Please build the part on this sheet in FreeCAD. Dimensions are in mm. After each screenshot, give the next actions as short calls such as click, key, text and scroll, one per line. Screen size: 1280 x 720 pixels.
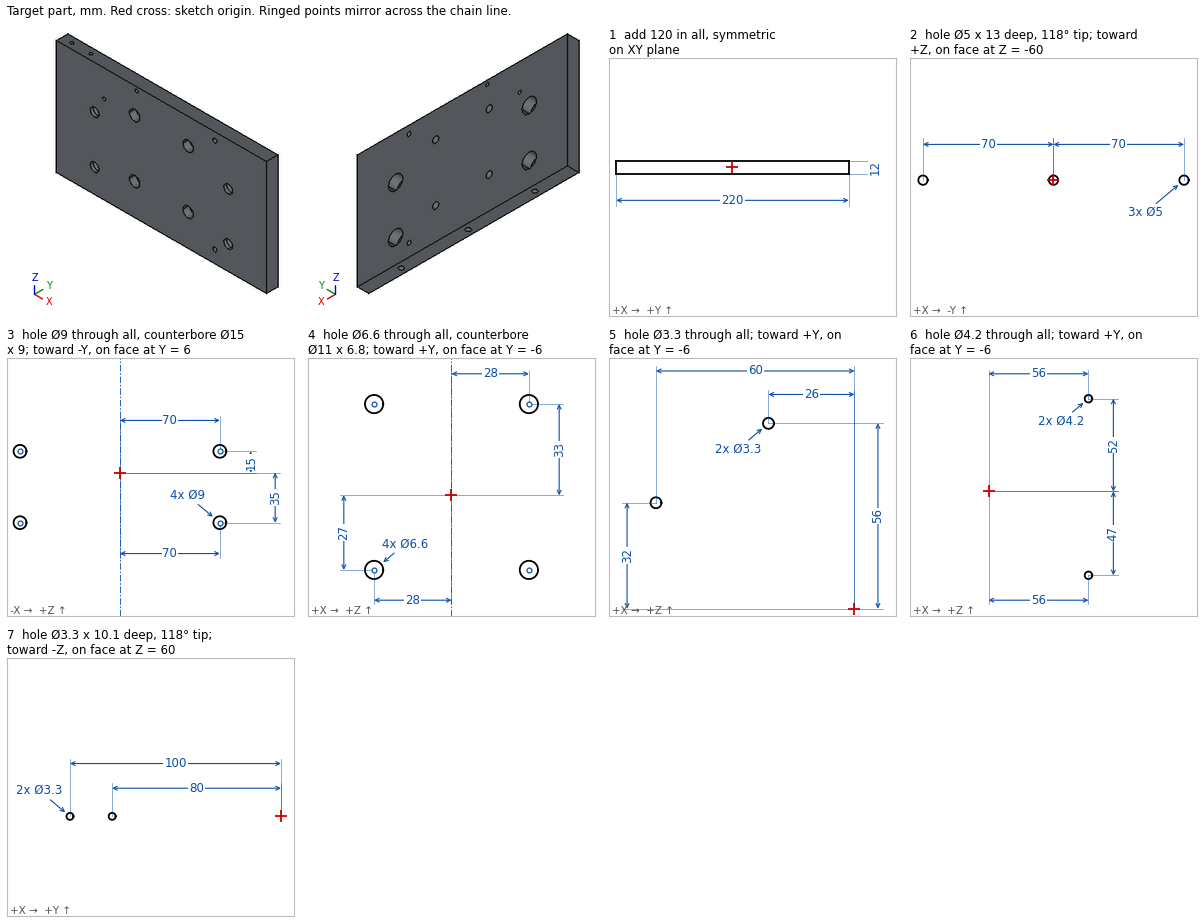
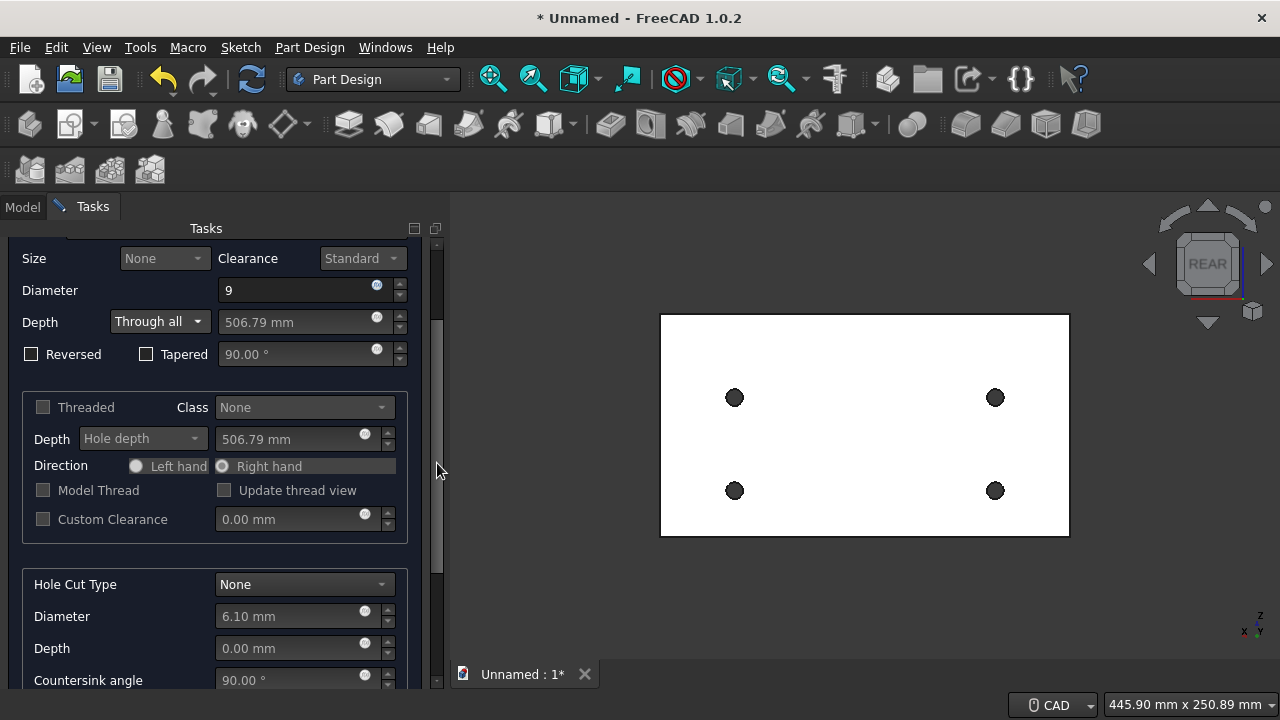
click(306, 584)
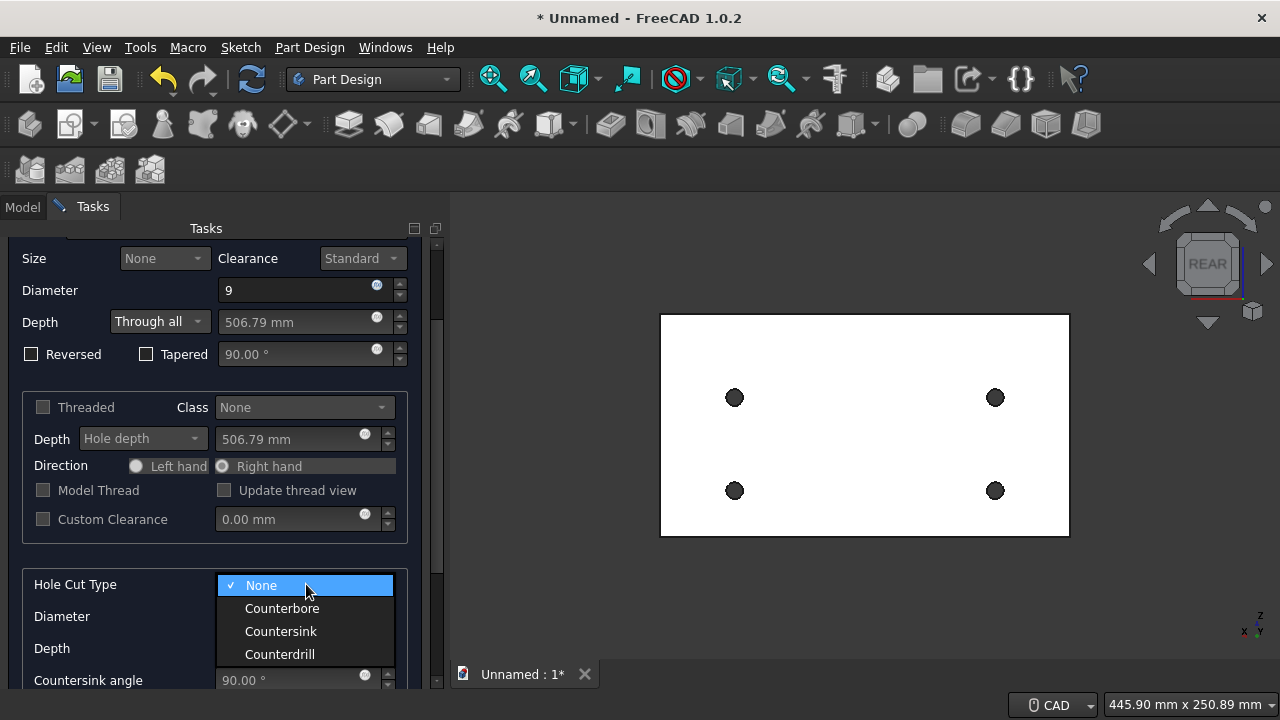
click(304, 608)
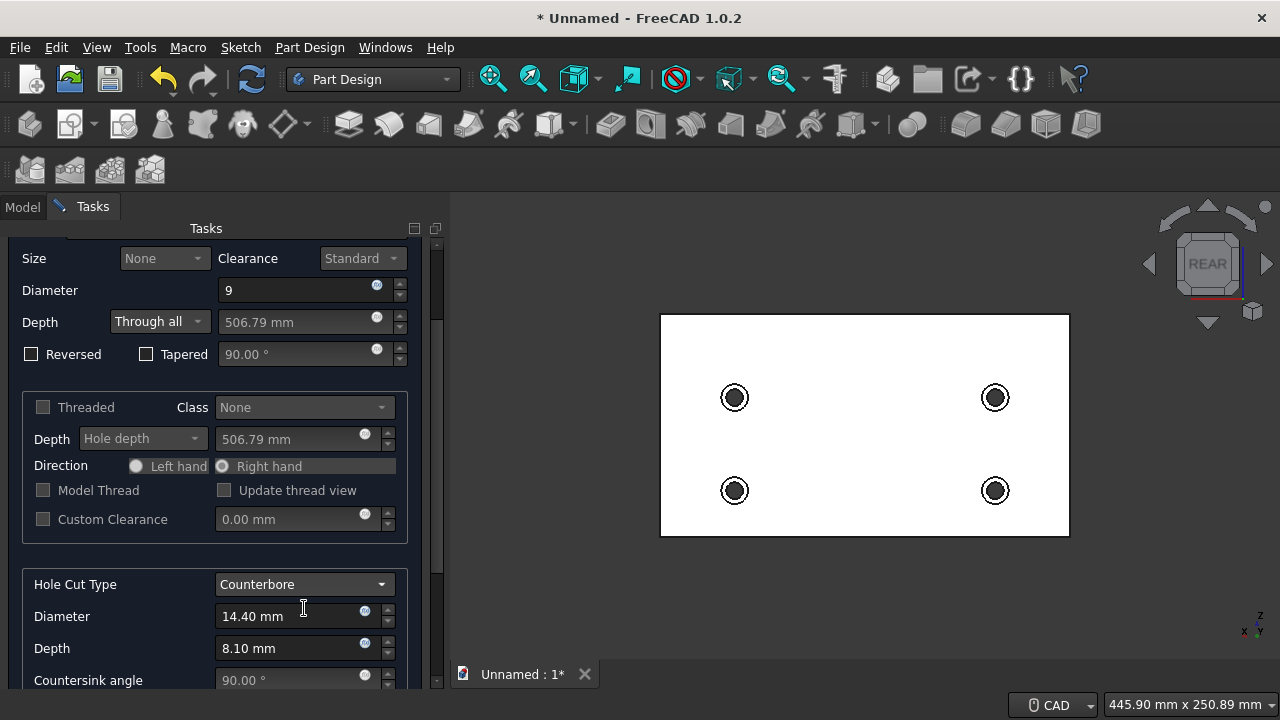
triple_click(298, 616)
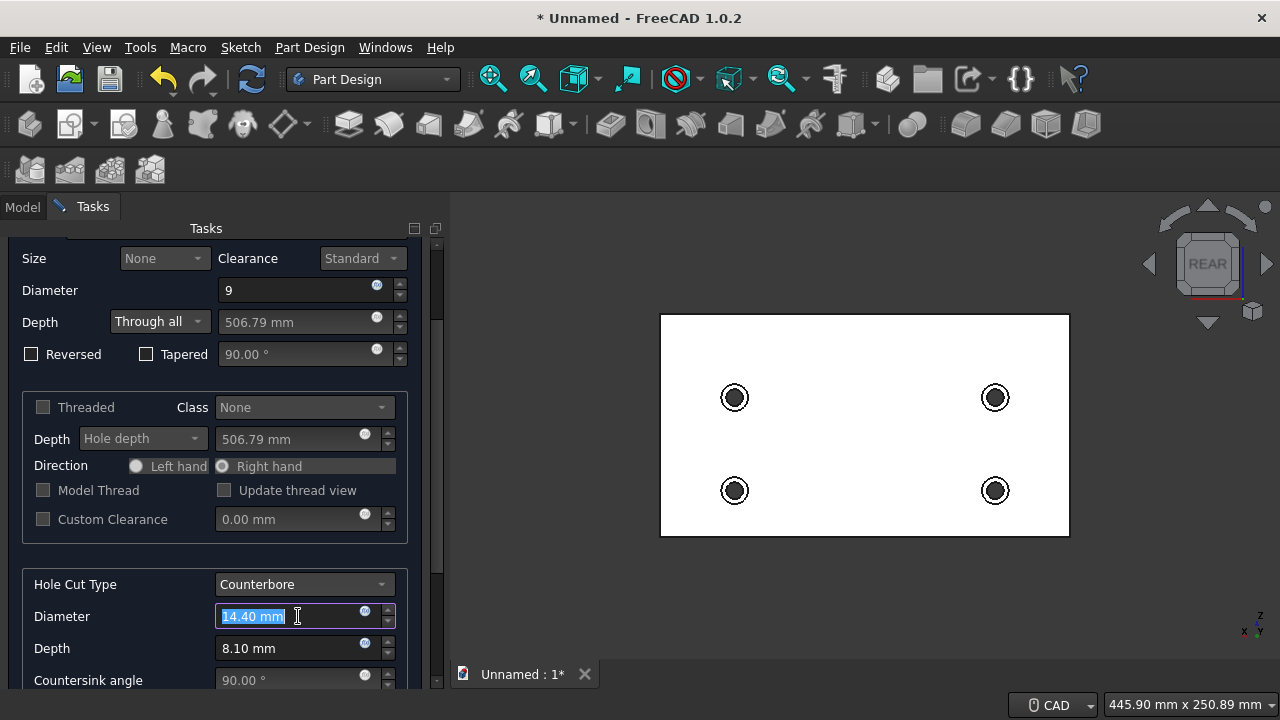
text(15)
key(Tab)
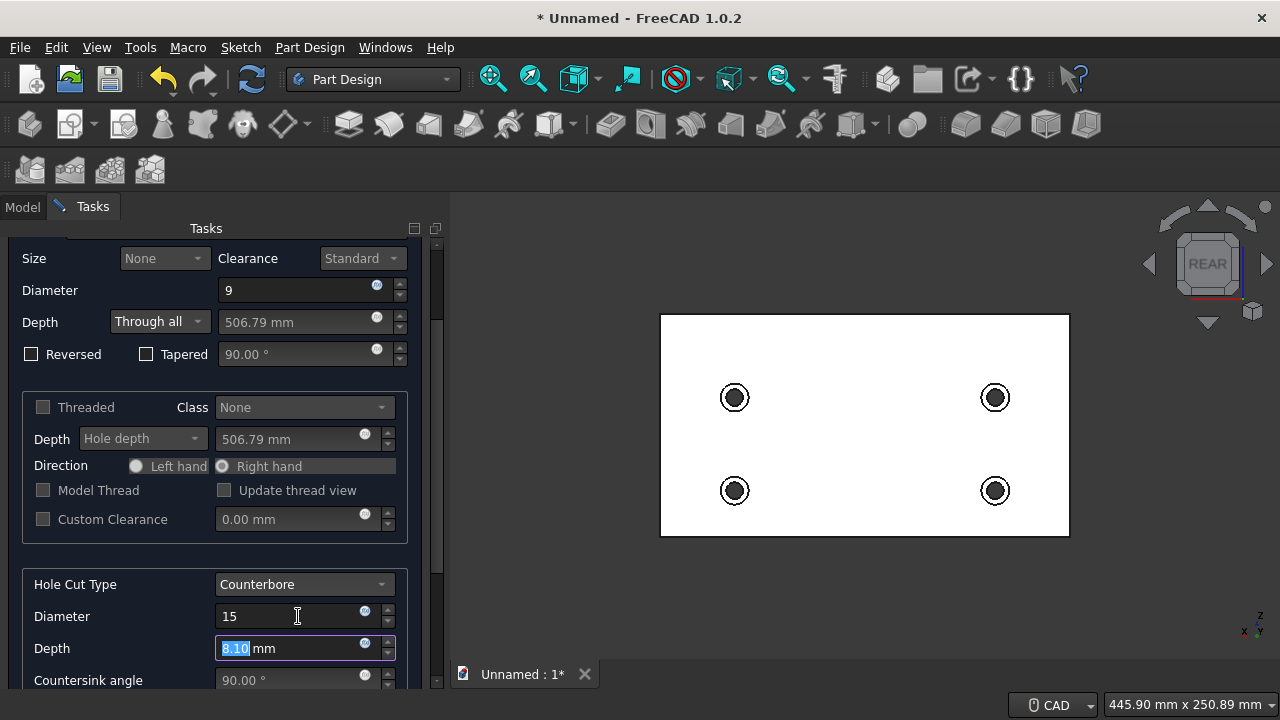
text(9)
key(Tab)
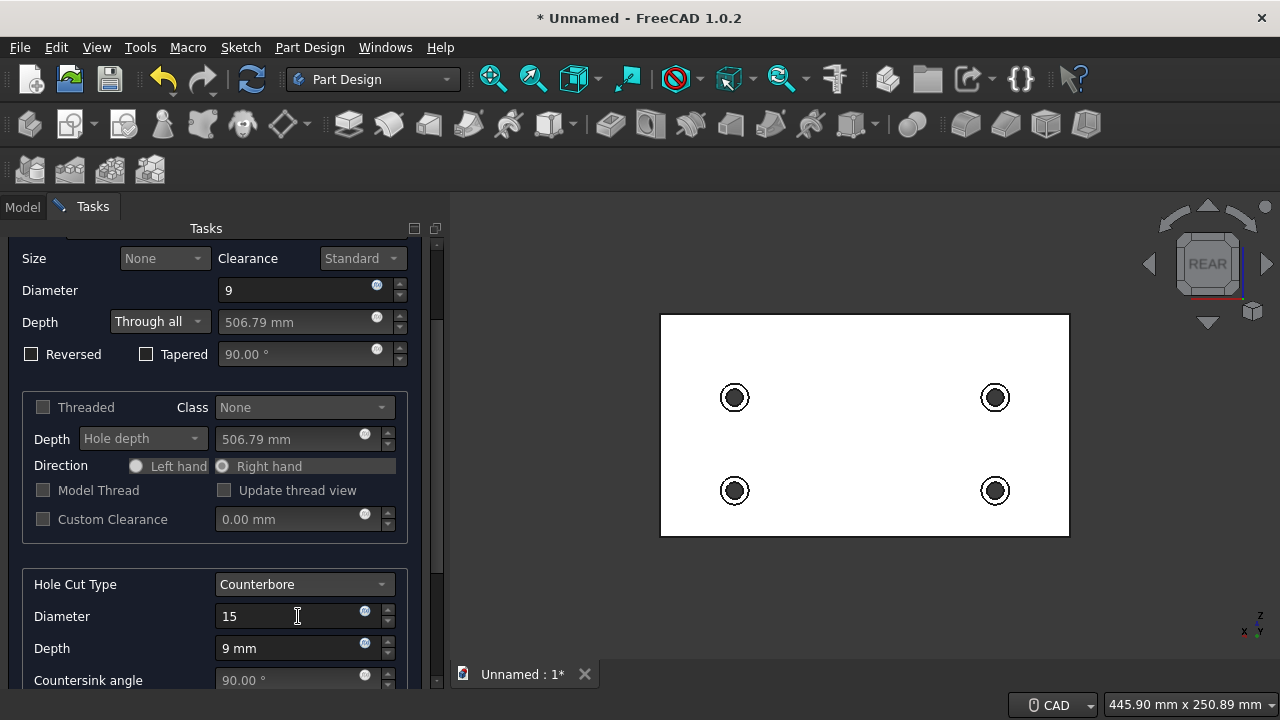
scroll(437, 463, up, 3)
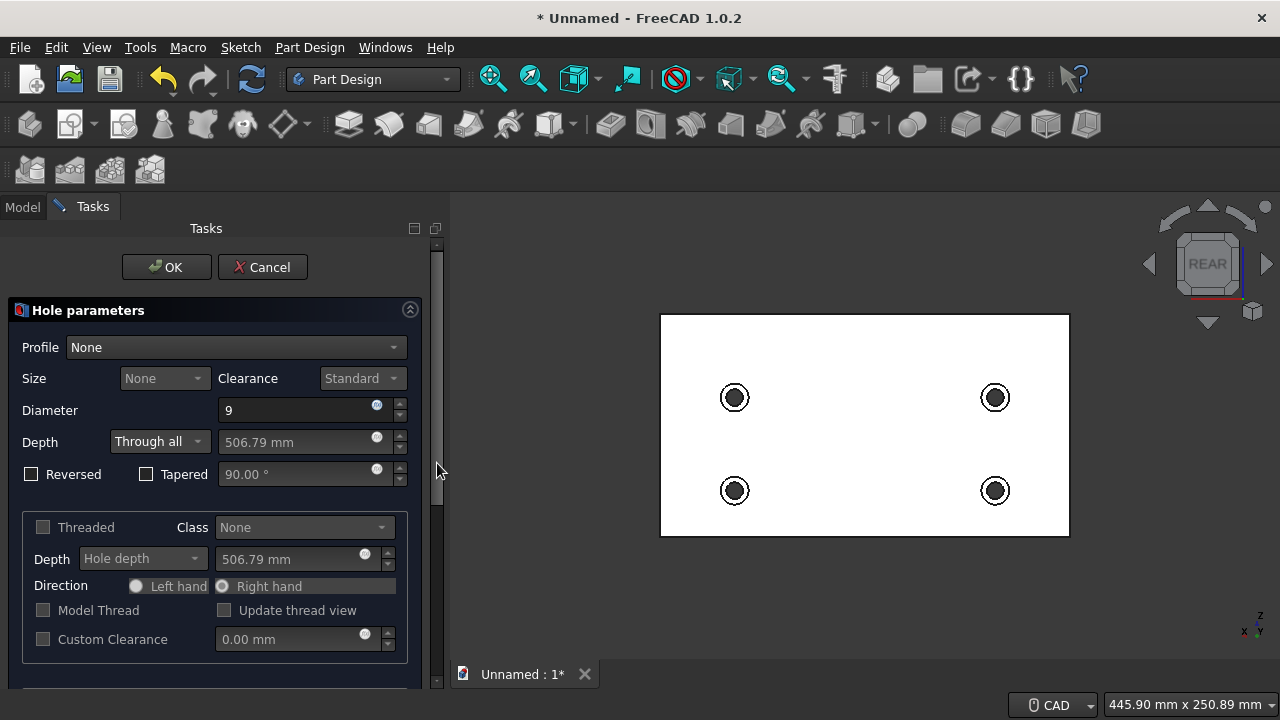
click(167, 267)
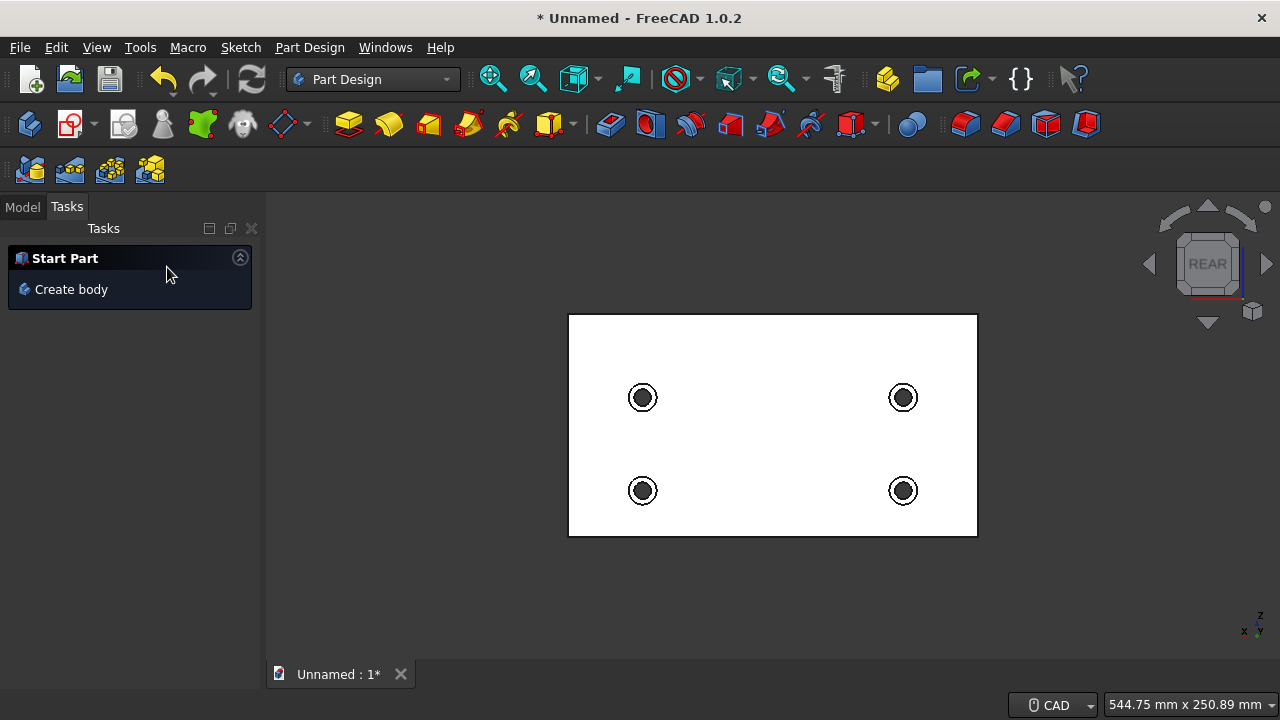
key(0)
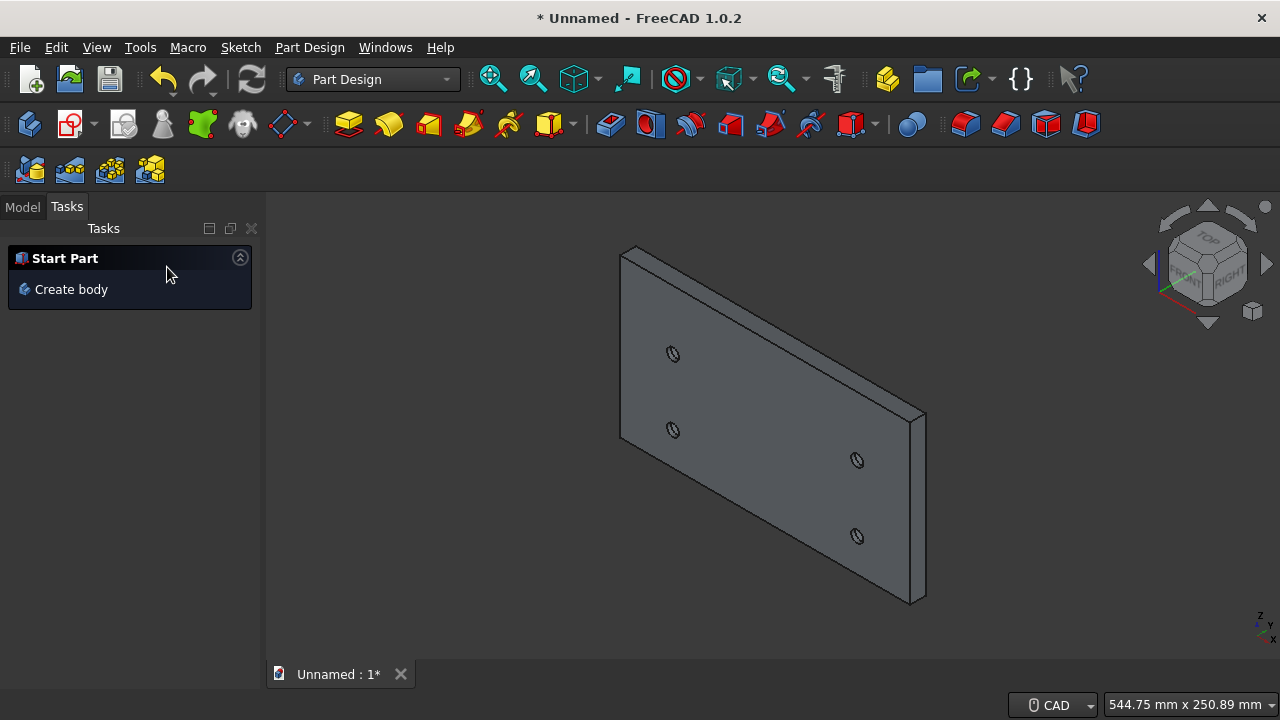
click(765, 429)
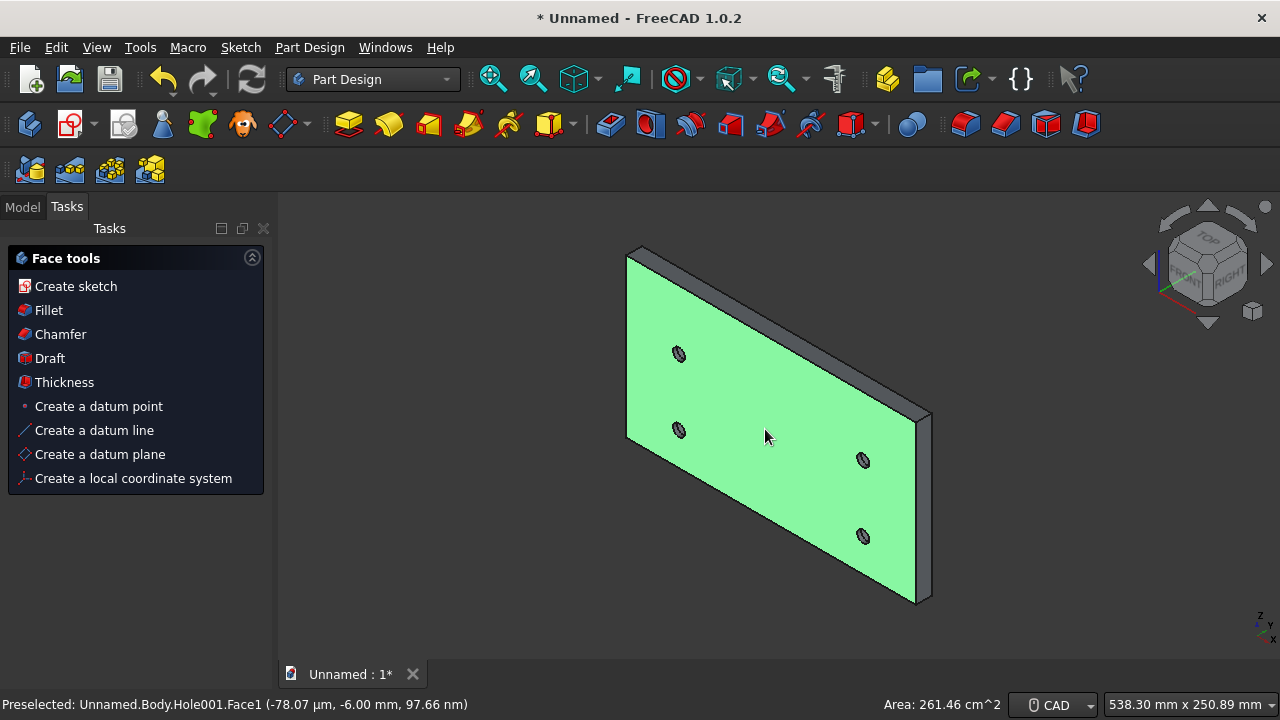
click(70, 124)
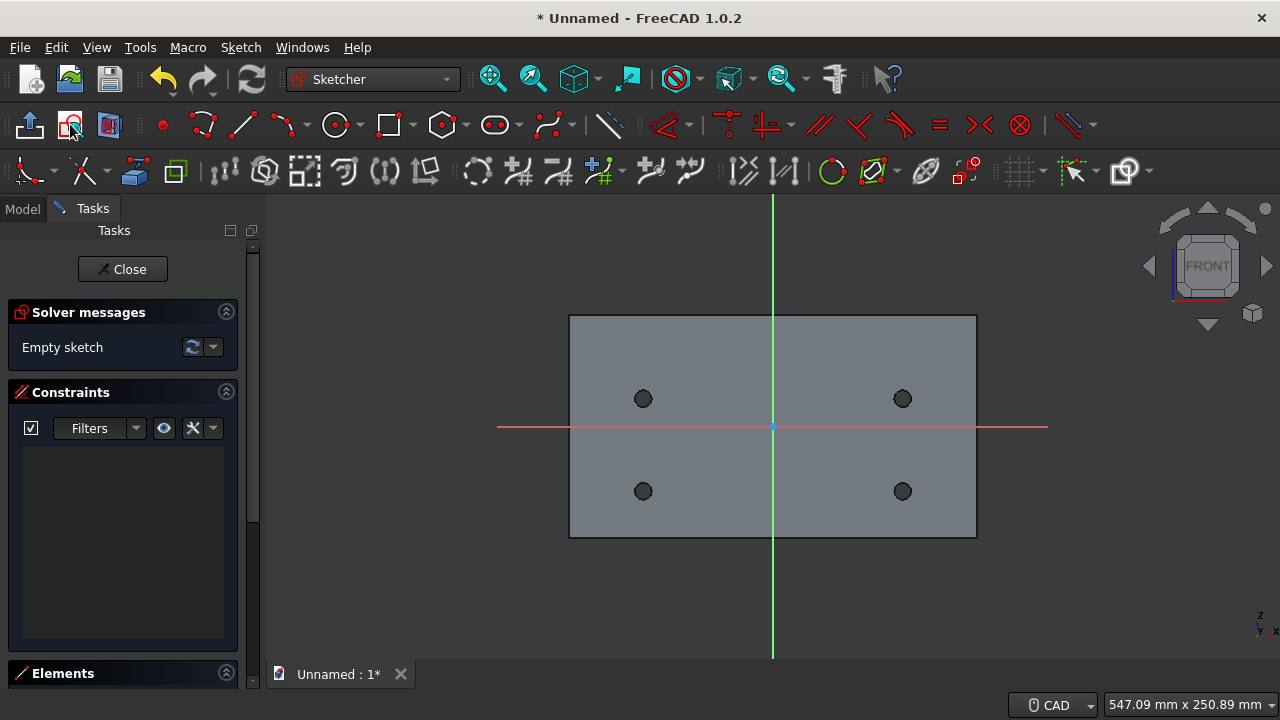
scroll(829, 416, up, 4)